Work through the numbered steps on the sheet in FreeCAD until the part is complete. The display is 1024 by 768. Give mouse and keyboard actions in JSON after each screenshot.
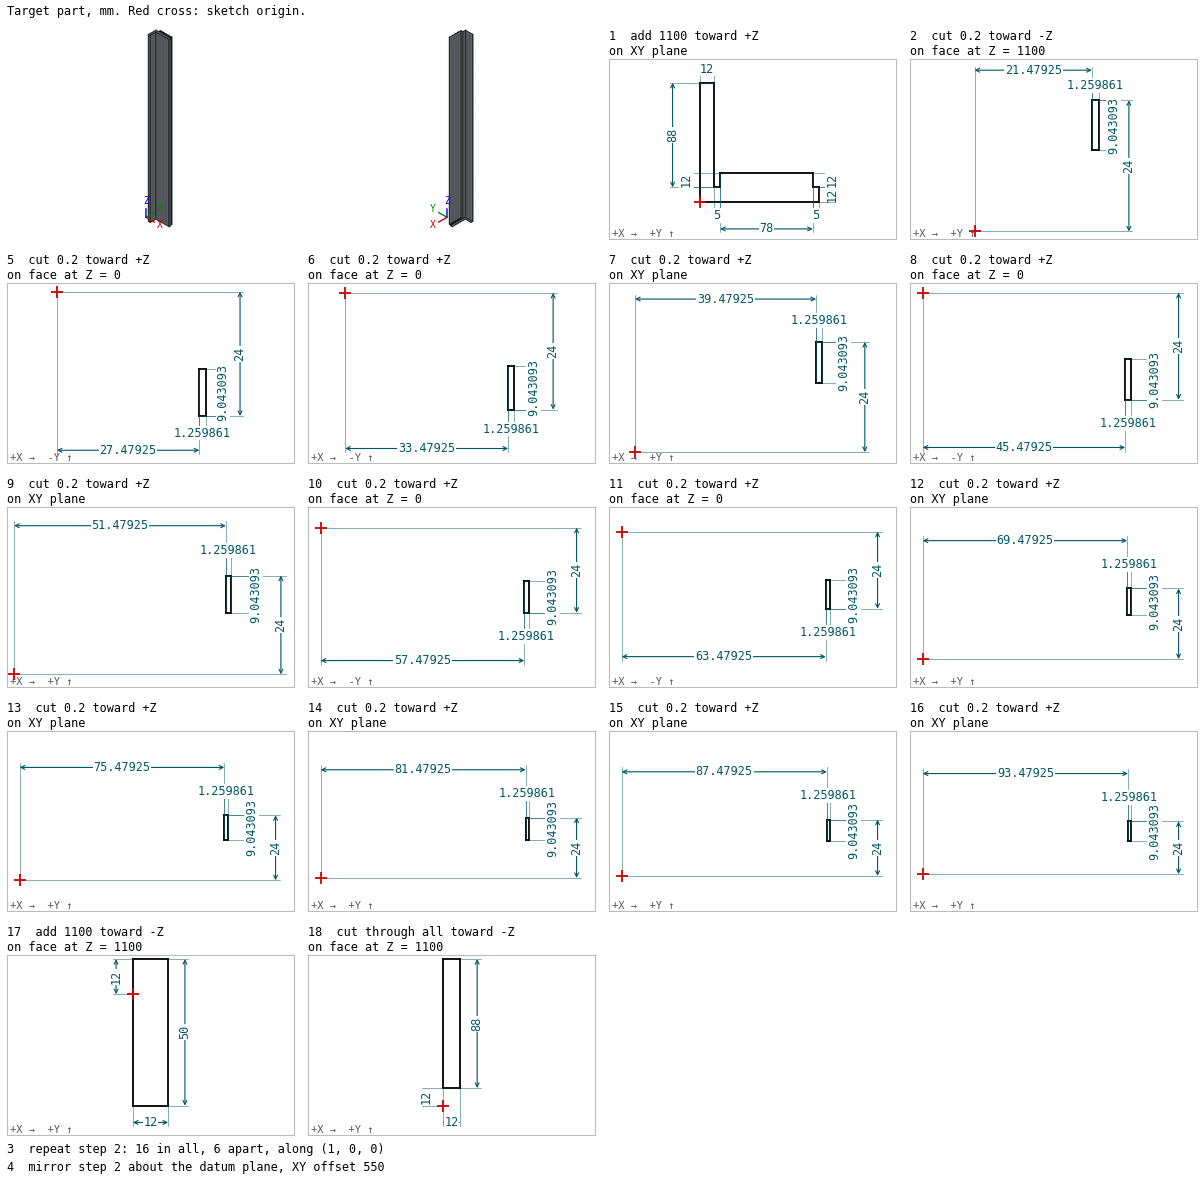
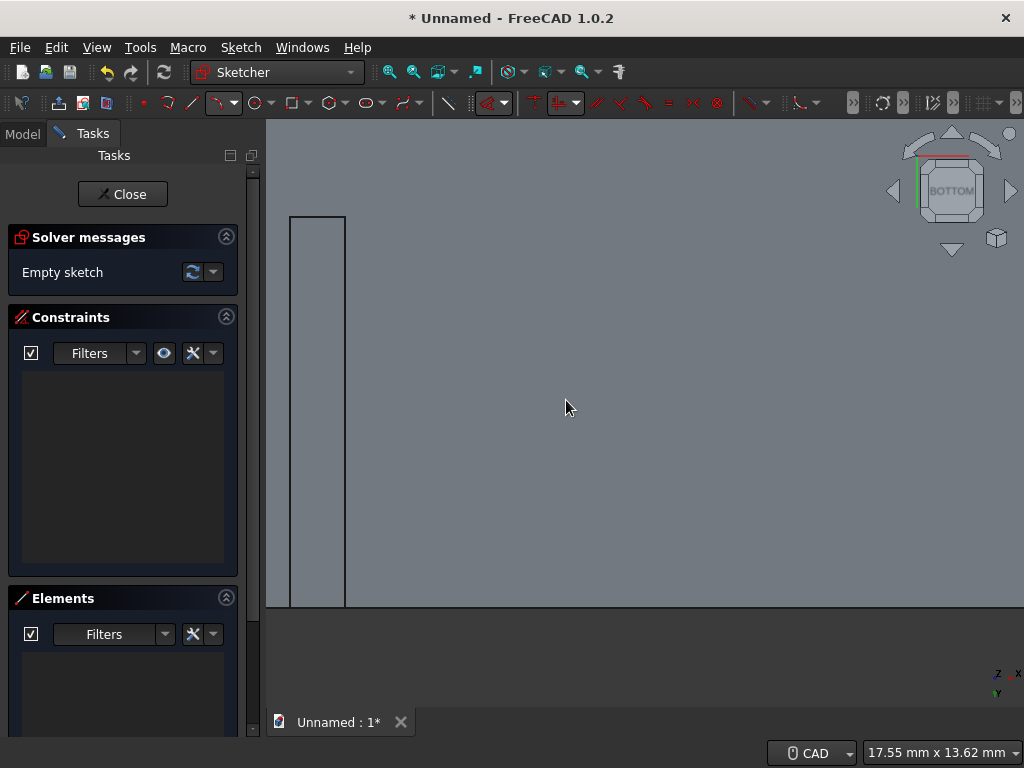
{"action": "key", "text": "g r"}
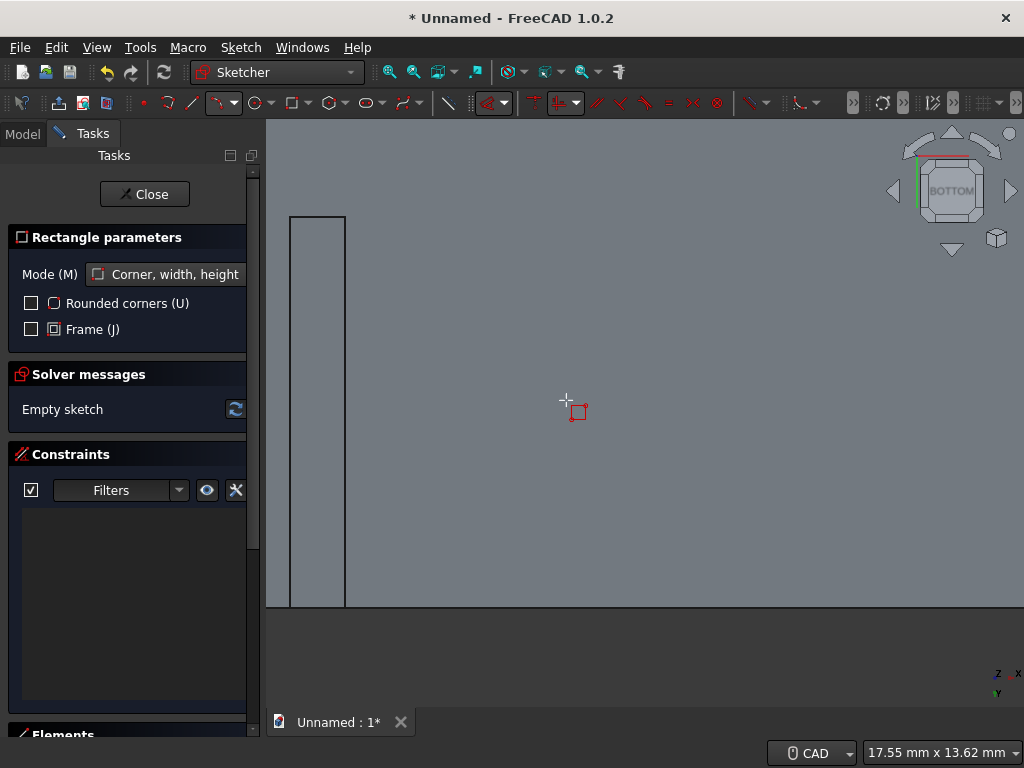
{"action": "left_click", "coordinate": [549, 217]}
{"action": "mouse_move", "coordinate": [604, 608]}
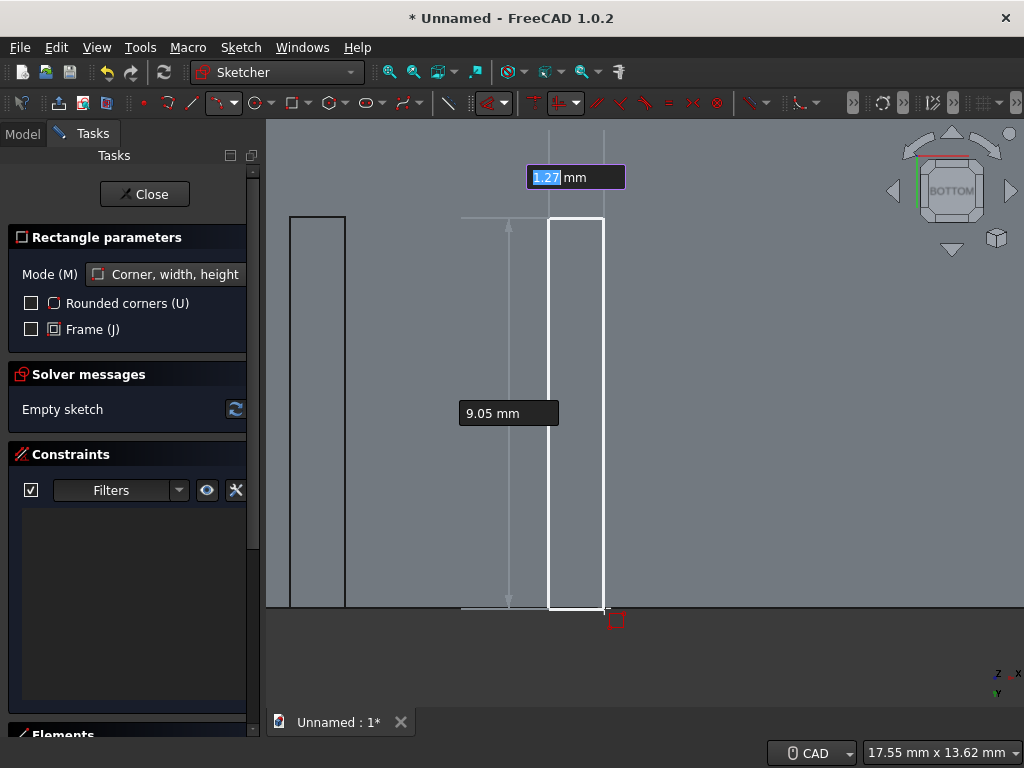
{"action": "type", "text": "1.259861"}
{"action": "key", "text": "Tab"}
{"action": "type", "text": "9.043093"}
{"action": "key", "text": "Return"}
{"action": "key", "text": "Escape"}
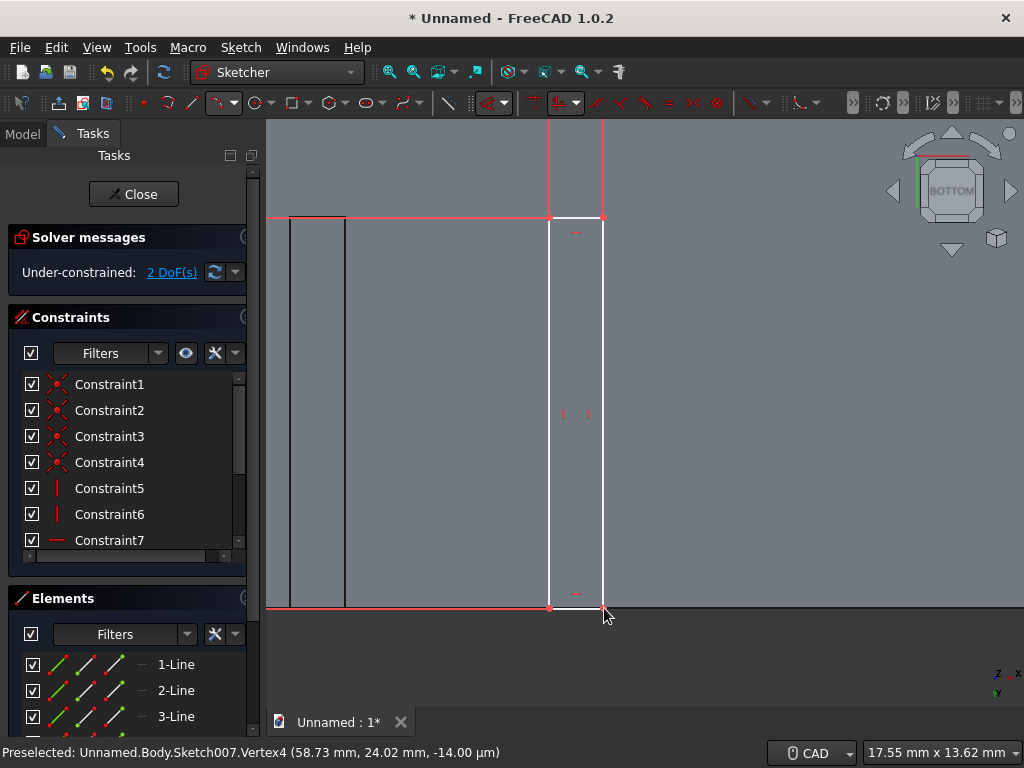
{"action": "left_click", "coordinate": [549, 609]}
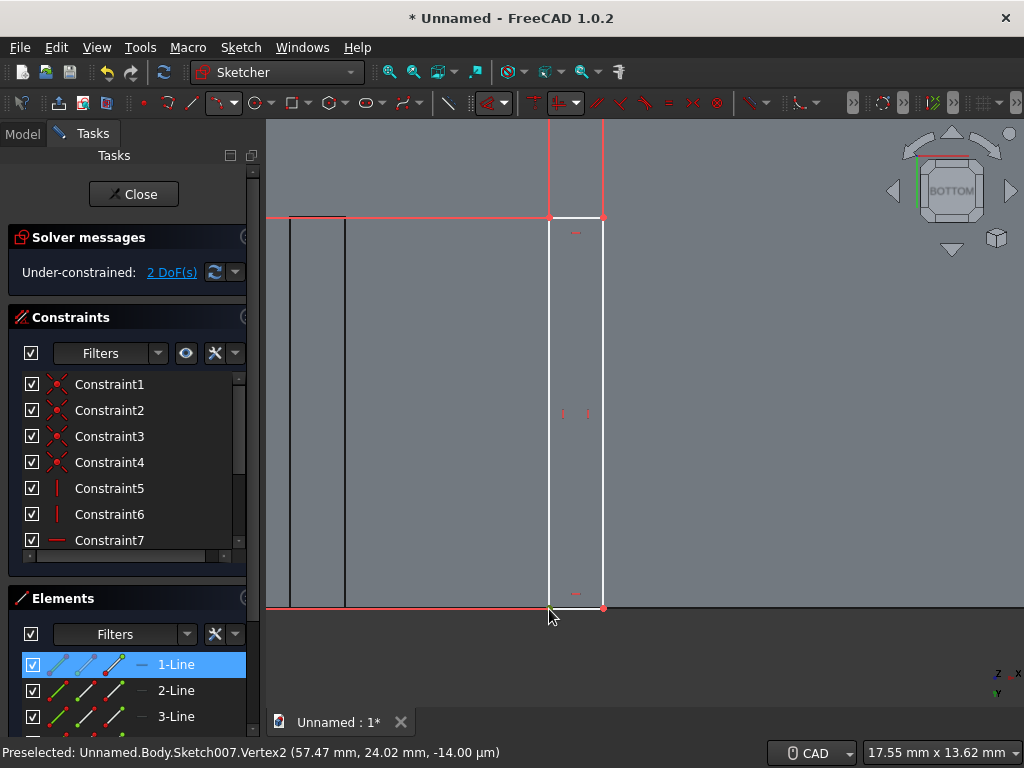
{"action": "key", "text": "i"}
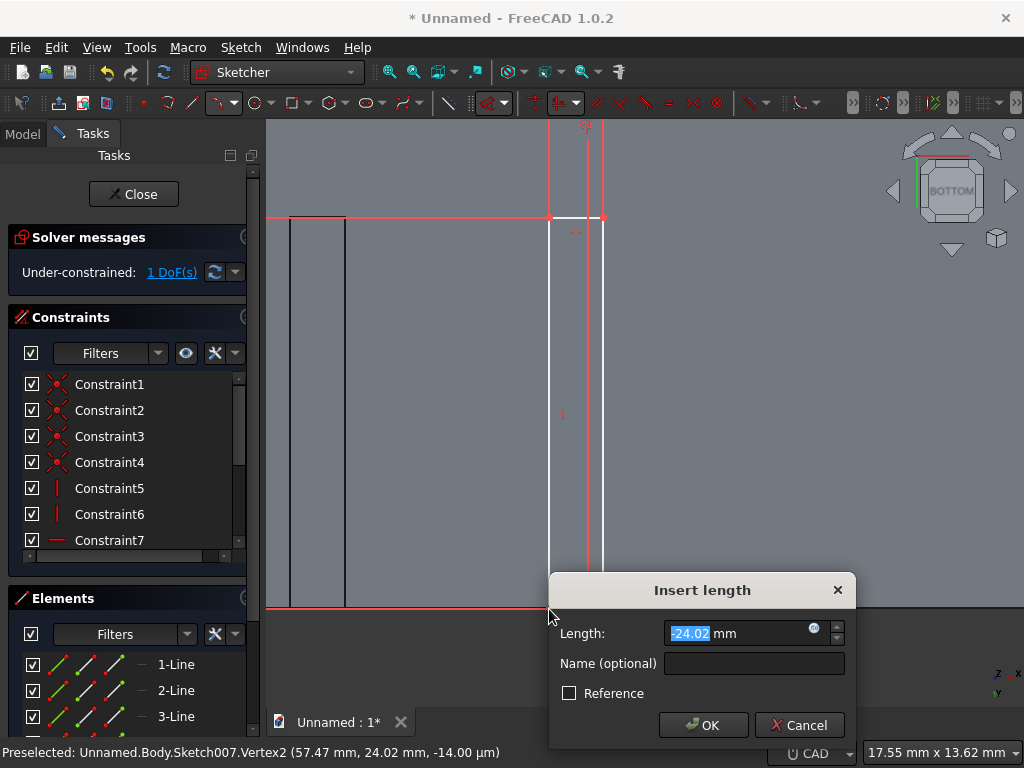
{"action": "type", "text": "-24"}
{"action": "key", "text": "Return"}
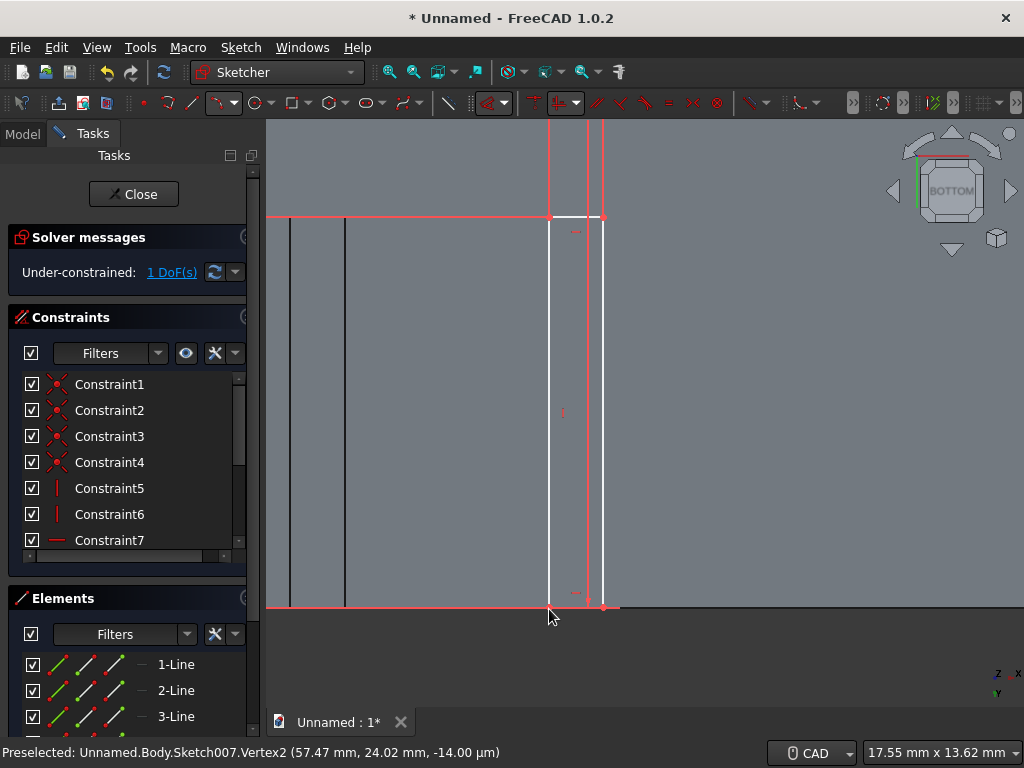
{"action": "left_click", "coordinate": [549, 217]}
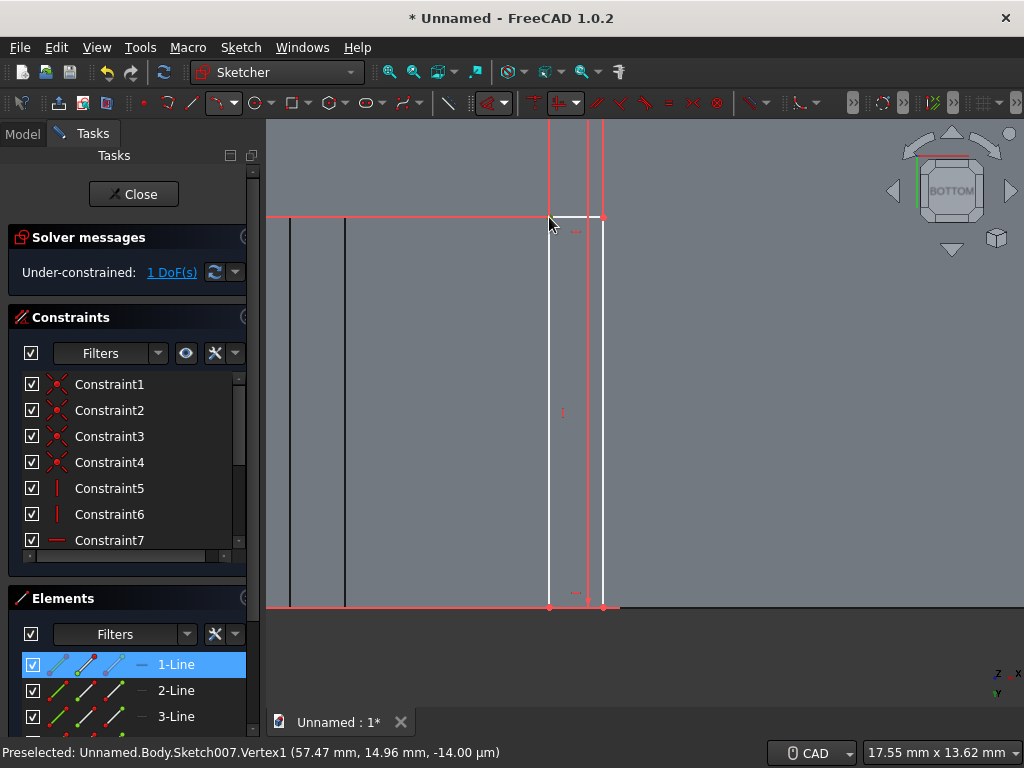
{"action": "key", "text": "l"}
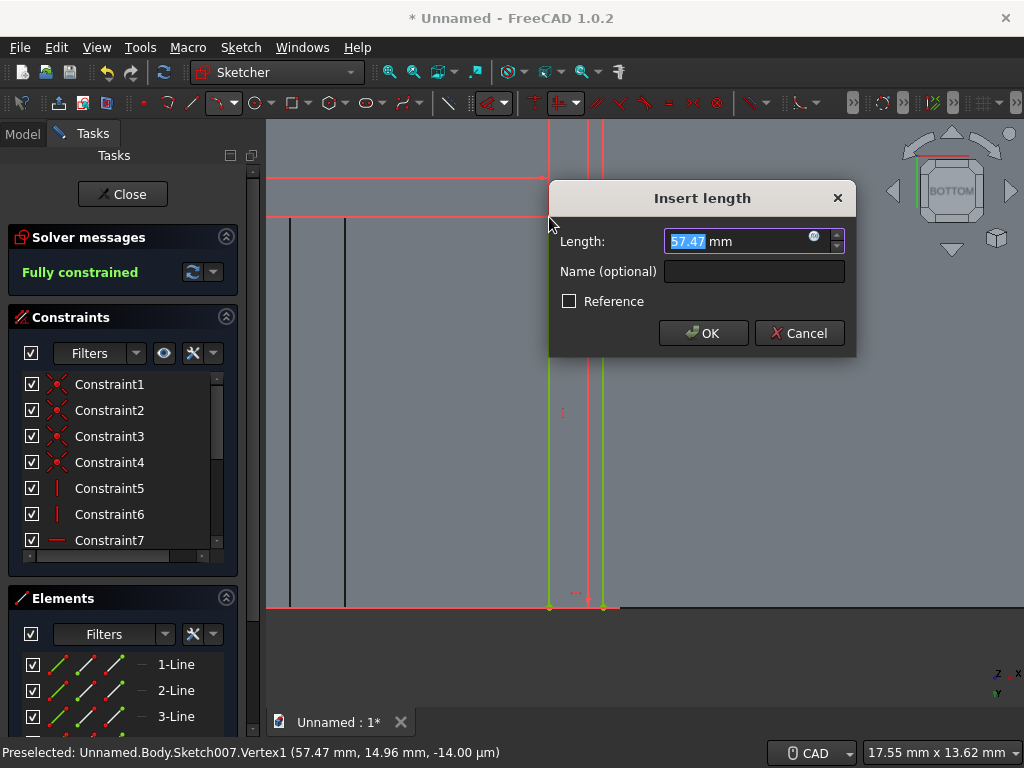
{"action": "type", "text": "57.47925"}
{"action": "key", "text": "Return"}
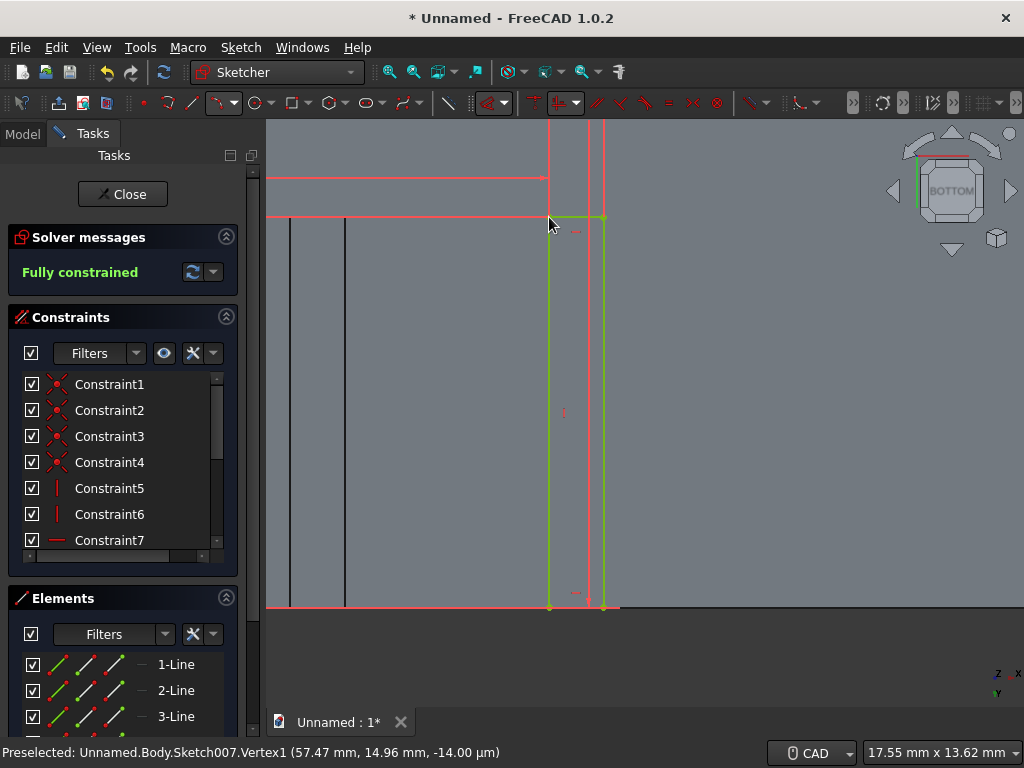
{"action": "left_click", "coordinate": [123, 194]}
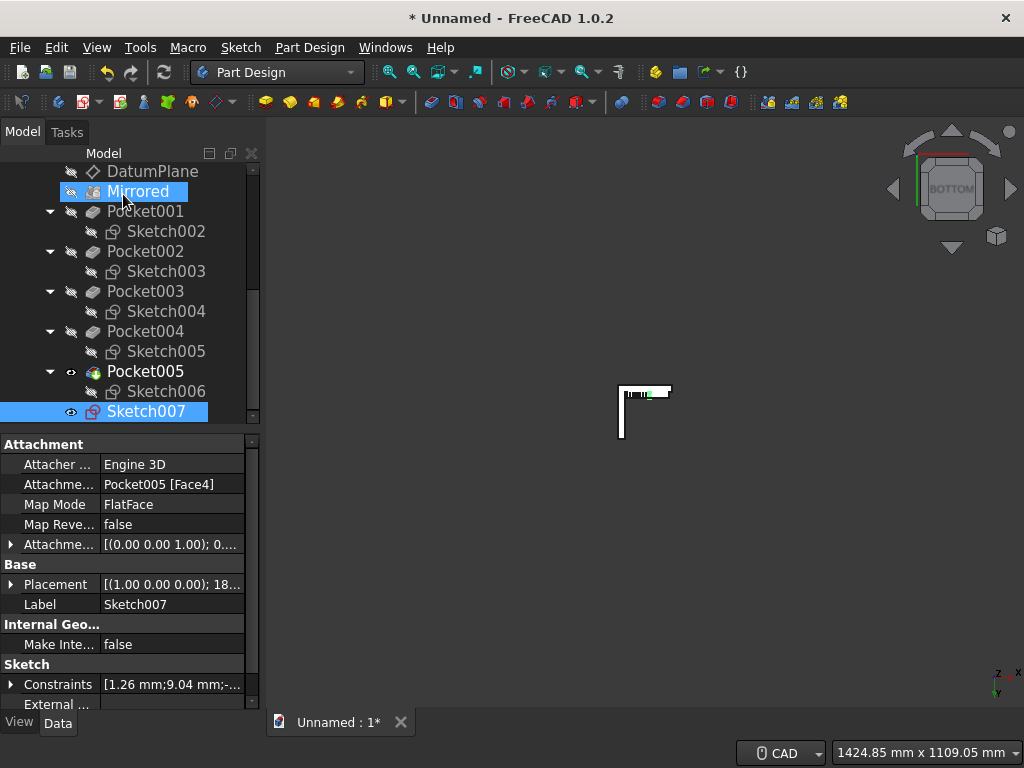
{"action": "left_click", "coordinate": [432, 102]}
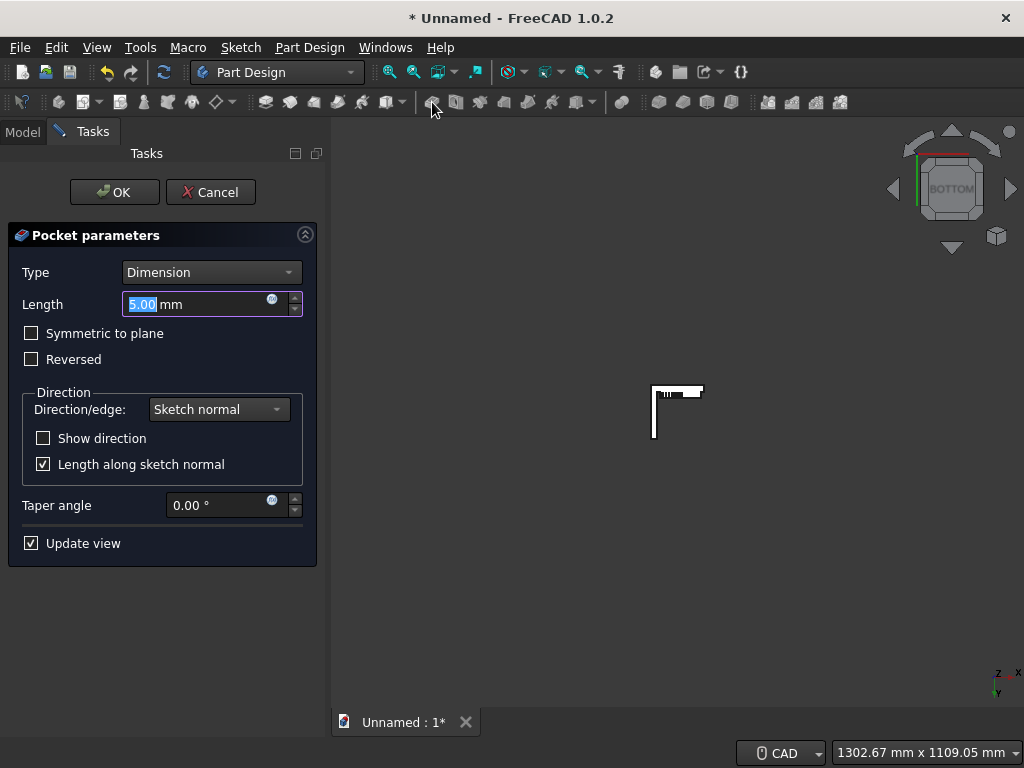
{"action": "type", "text": "0.2"}
{"action": "key", "text": "Tab"}